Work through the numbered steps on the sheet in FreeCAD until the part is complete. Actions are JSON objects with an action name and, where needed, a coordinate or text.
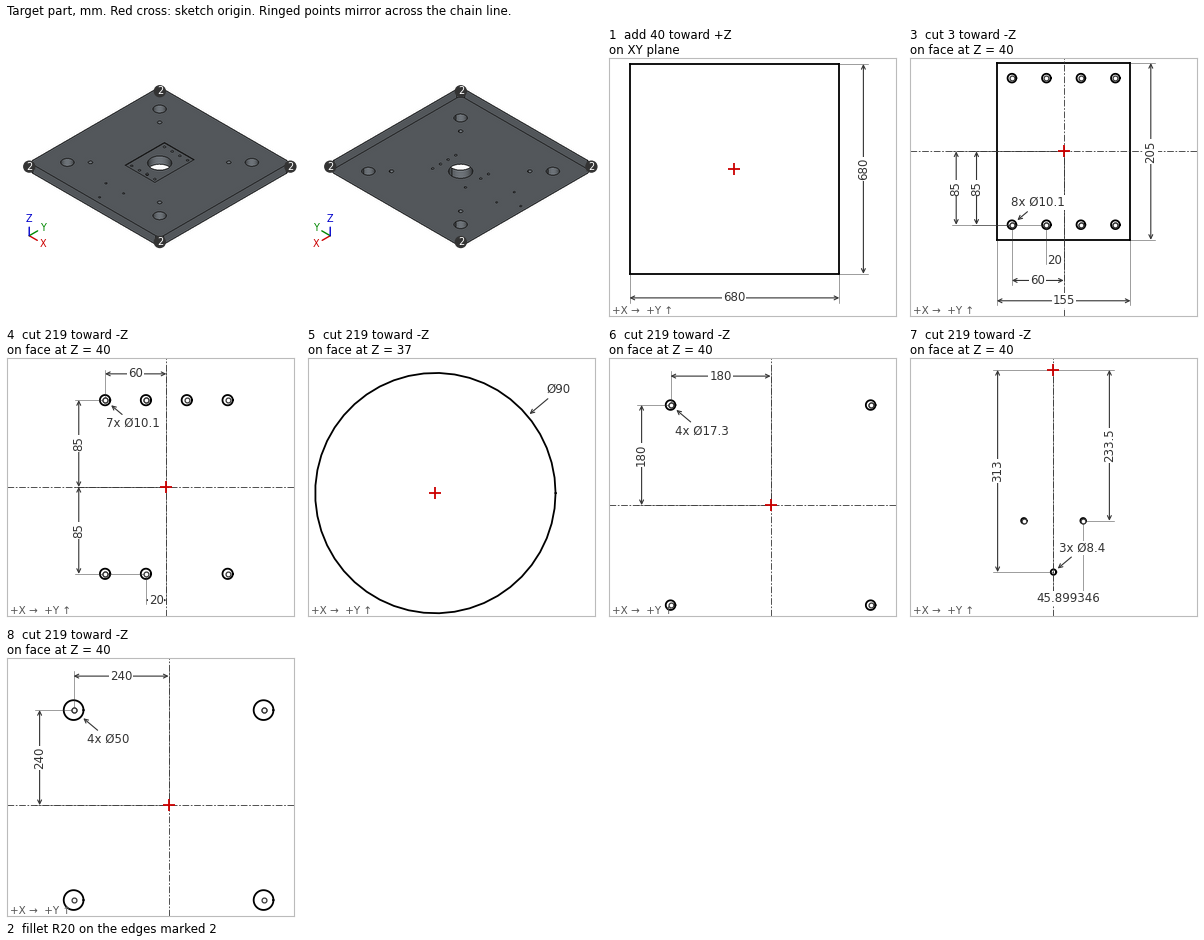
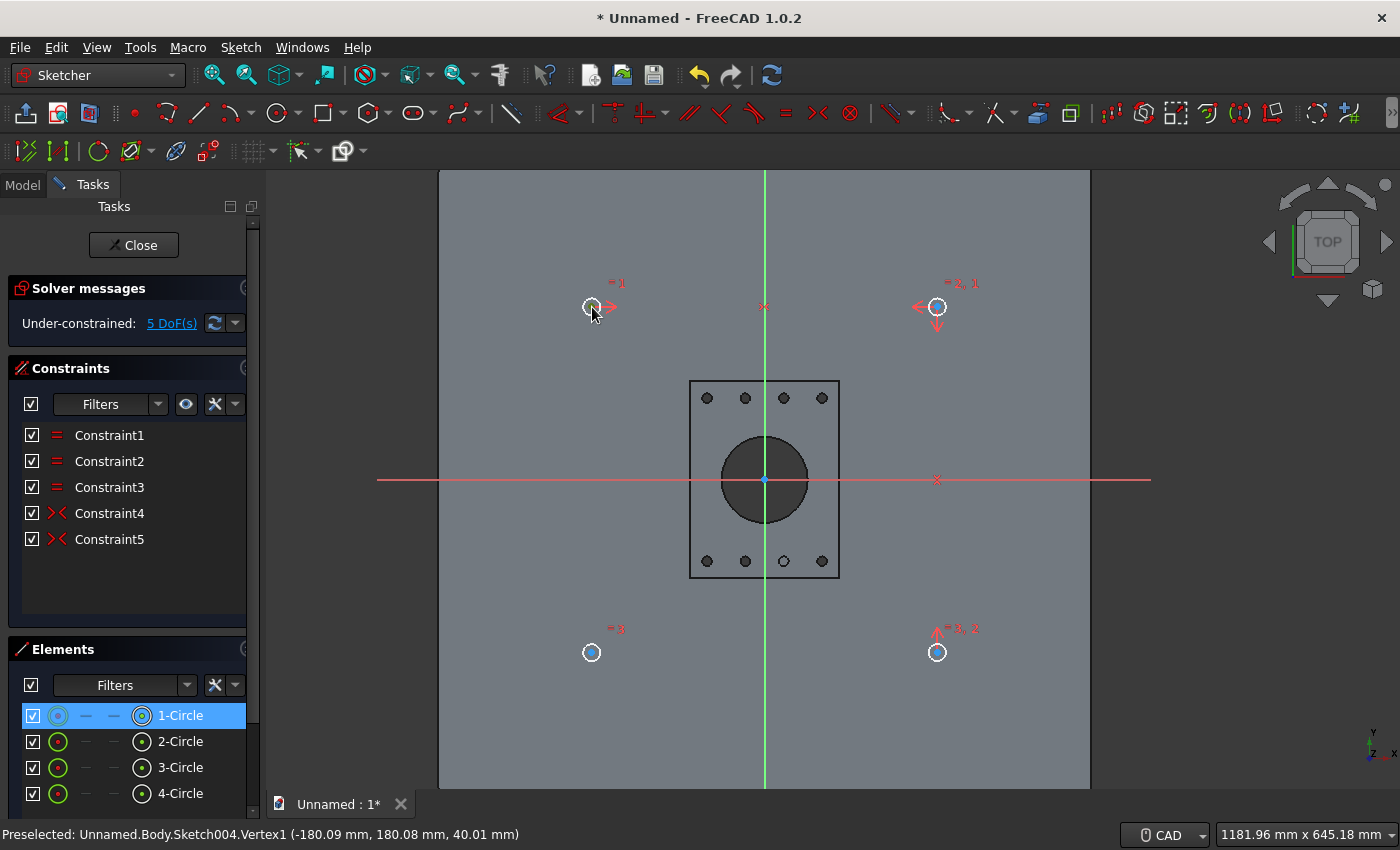
{"action": "left_click", "coordinate": [592, 653]}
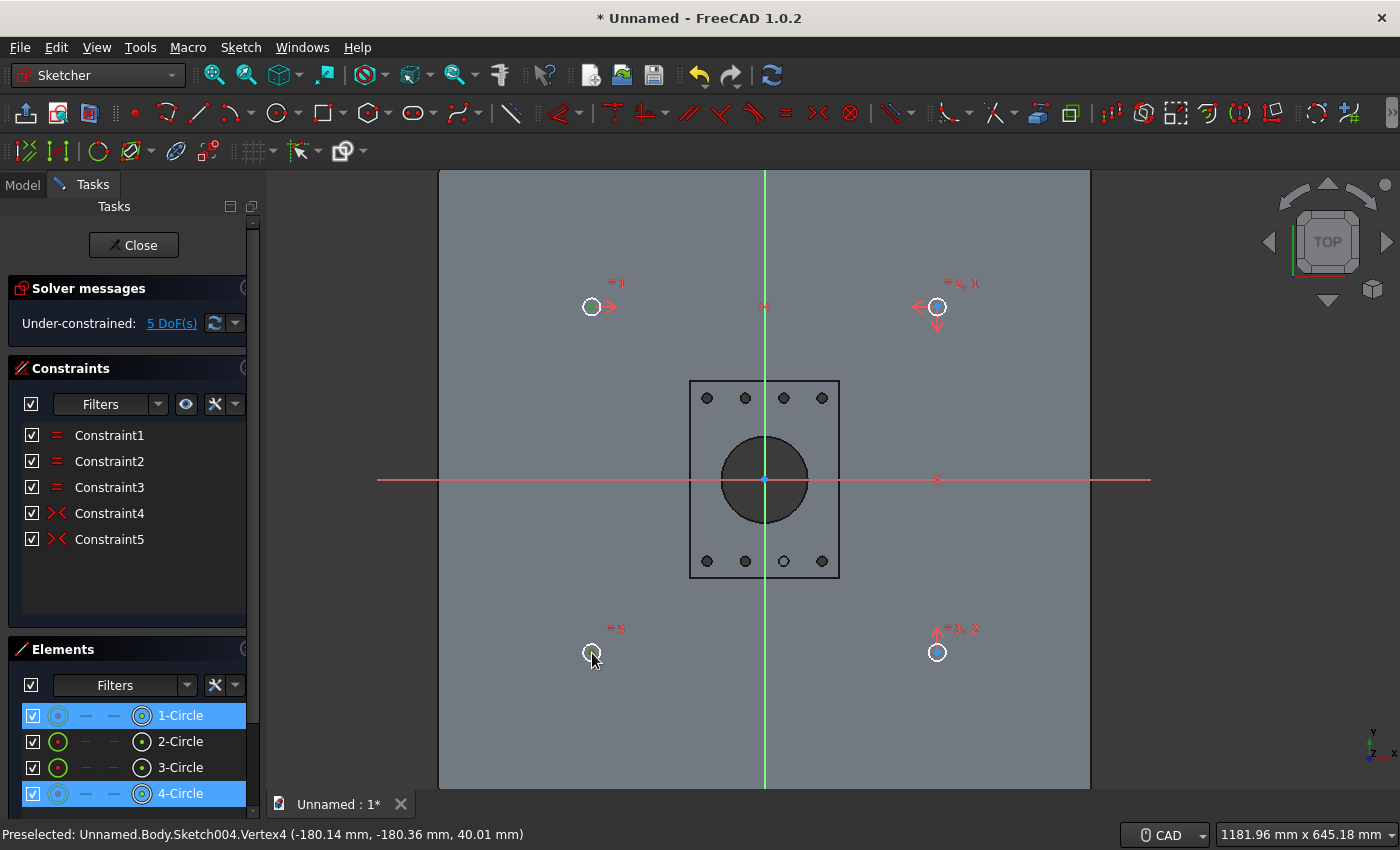
{"action": "left_click", "coordinate": [428, 480]}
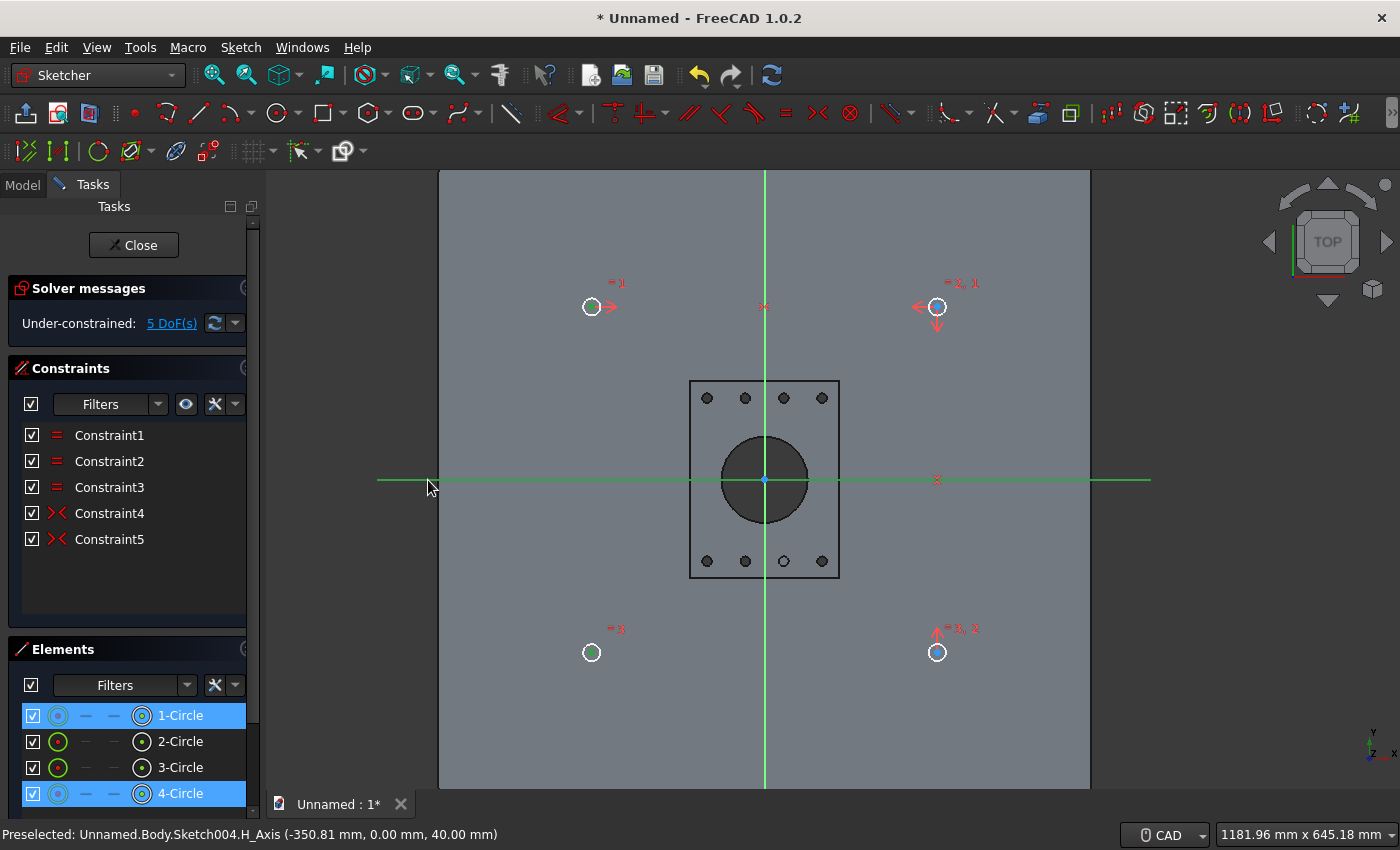
{"action": "left_click", "coordinate": [818, 114]}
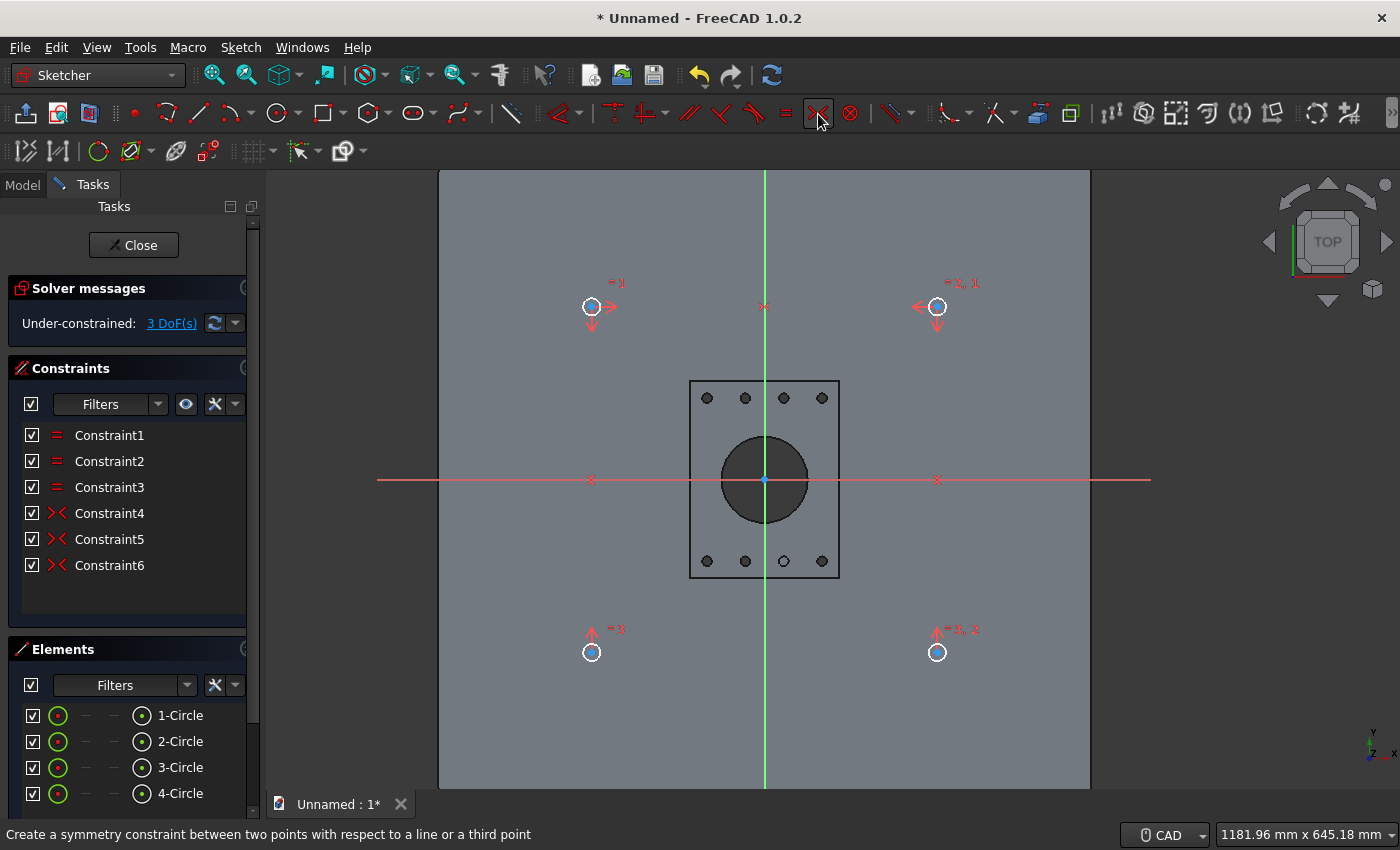
{"action": "left_click", "coordinate": [558, 114]}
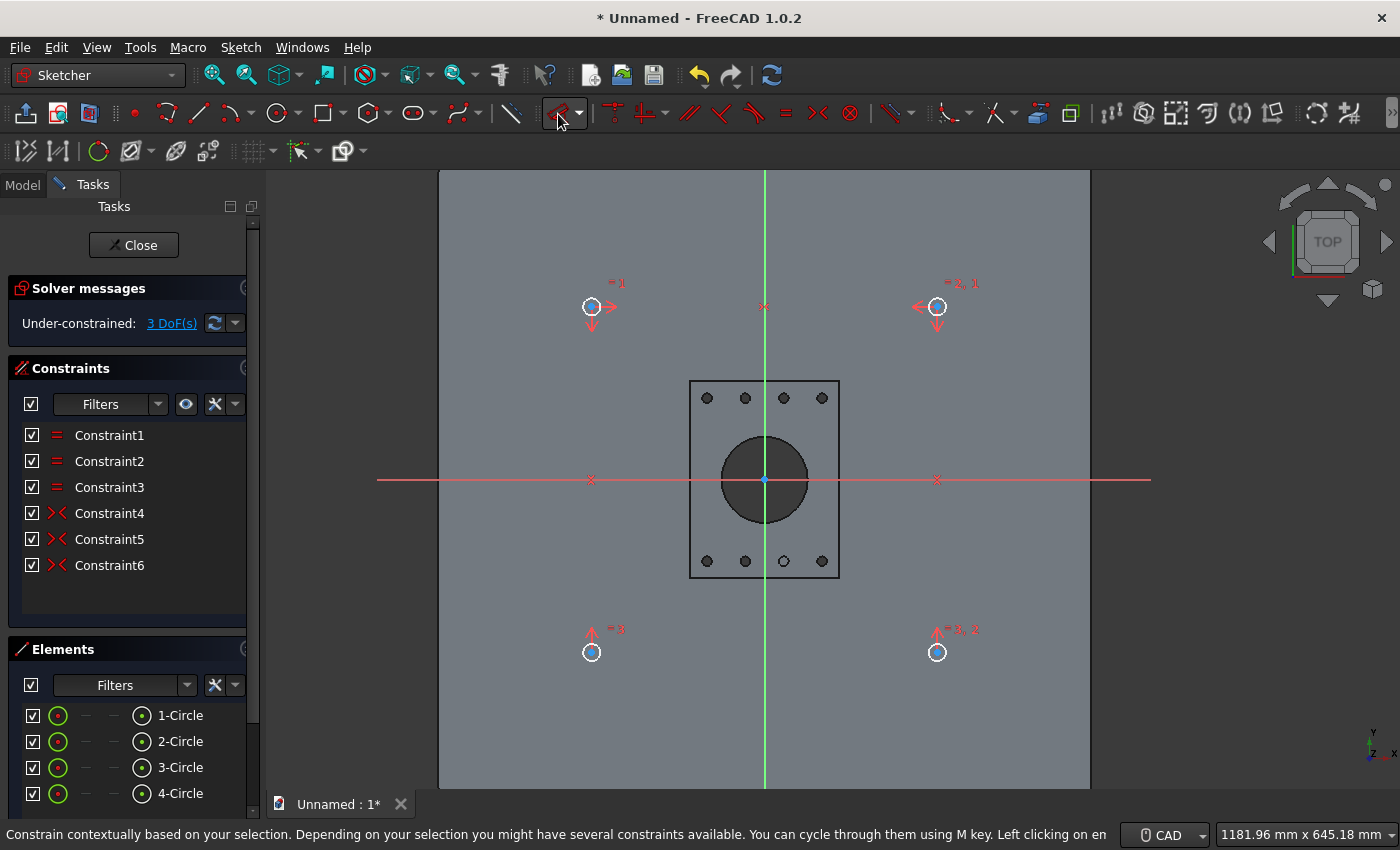
{"action": "scroll", "coordinate": [598, 313], "scroll_direction": "up", "scroll_amount": 5}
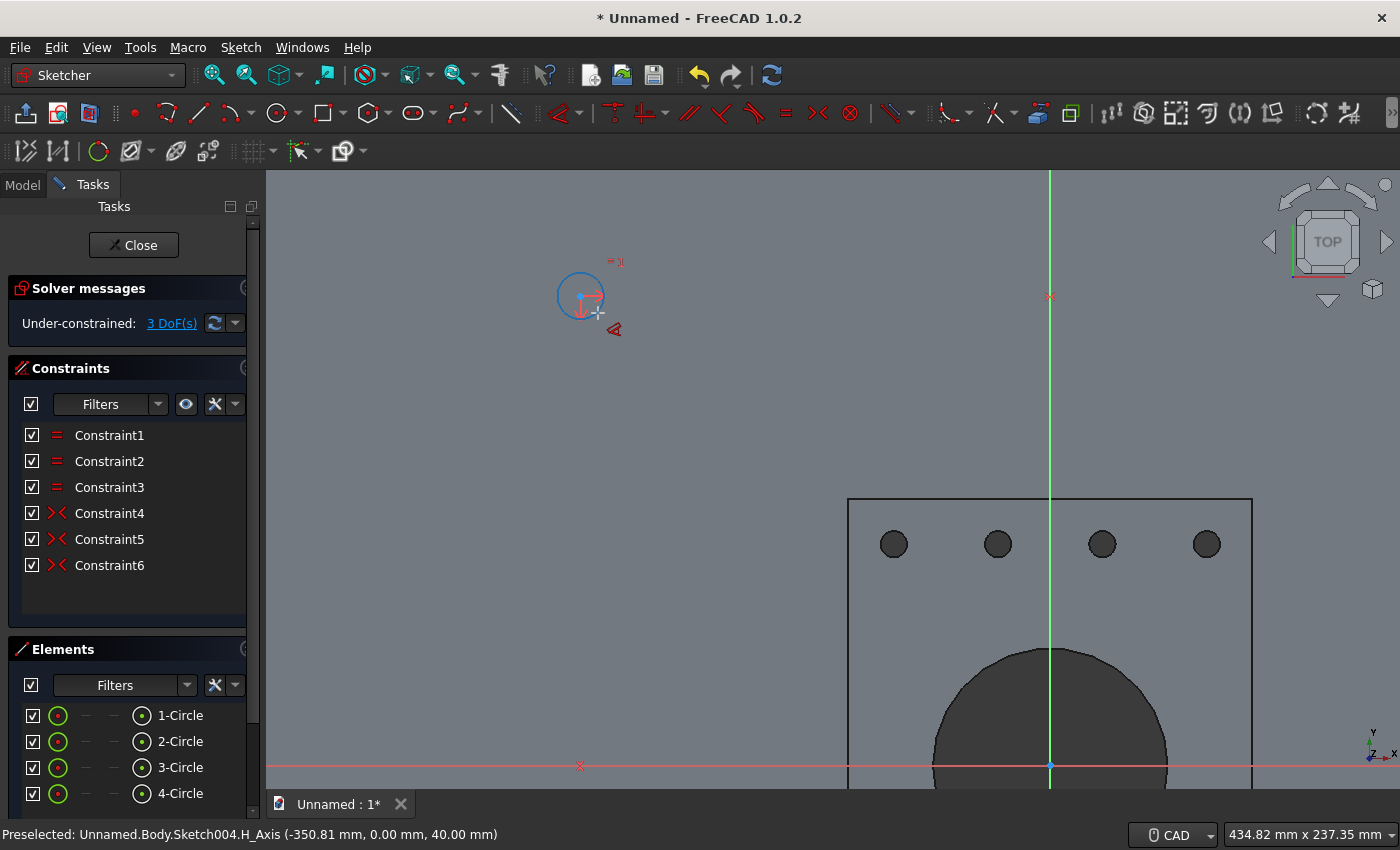
{"action": "left_click", "coordinate": [597, 312]}
{"action": "left_click", "coordinate": [620, 334]}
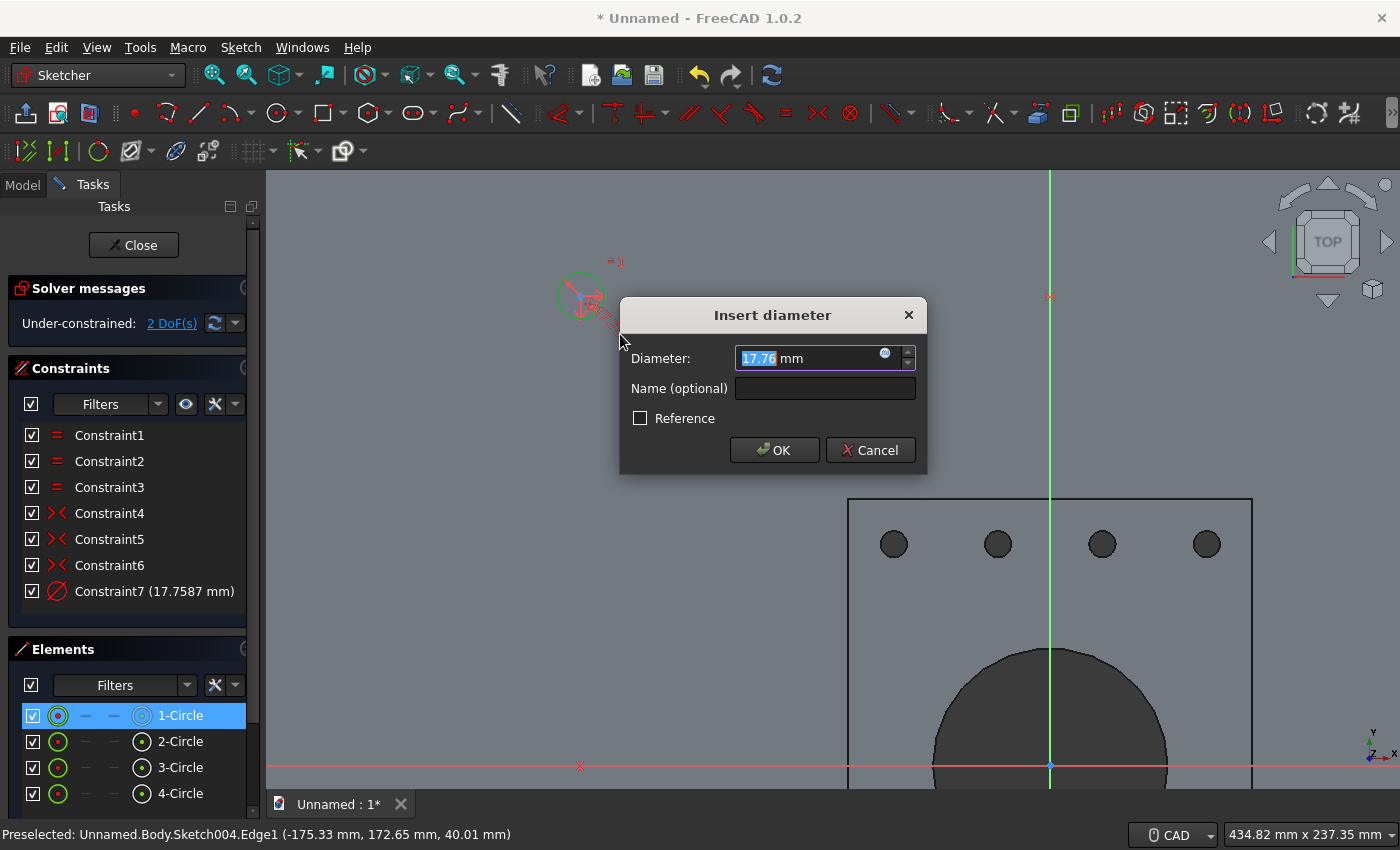
{"action": "type", "text": "17.3"}
{"action": "key", "text": "Return"}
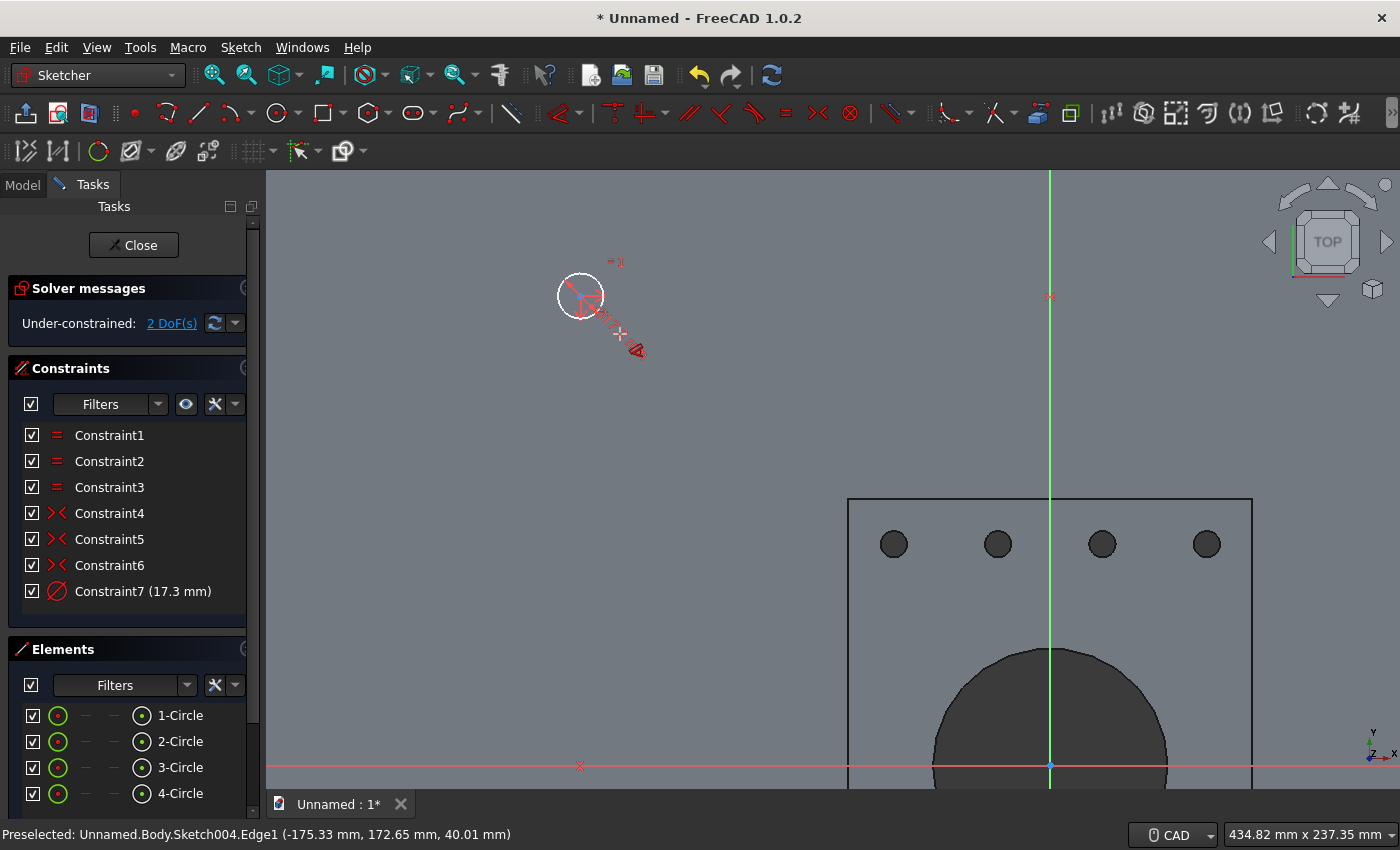
{"action": "left_click", "coordinate": [581, 296]}
{"action": "left_click", "coordinate": [815, 262]}